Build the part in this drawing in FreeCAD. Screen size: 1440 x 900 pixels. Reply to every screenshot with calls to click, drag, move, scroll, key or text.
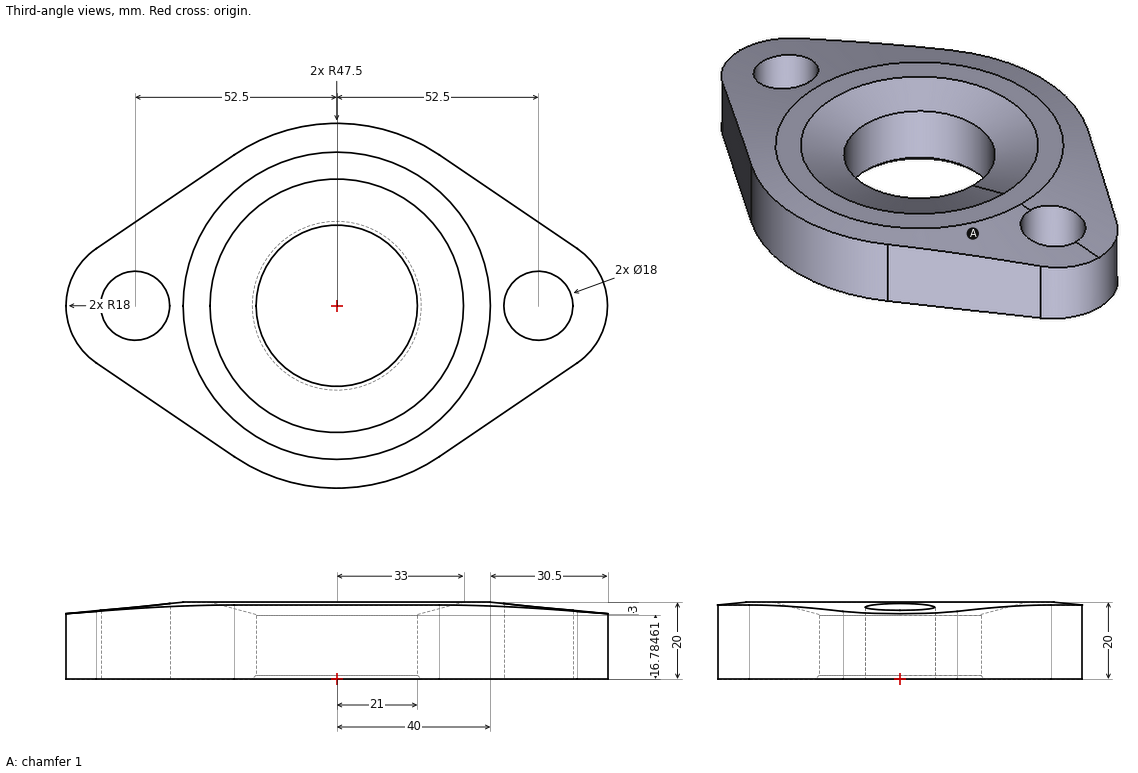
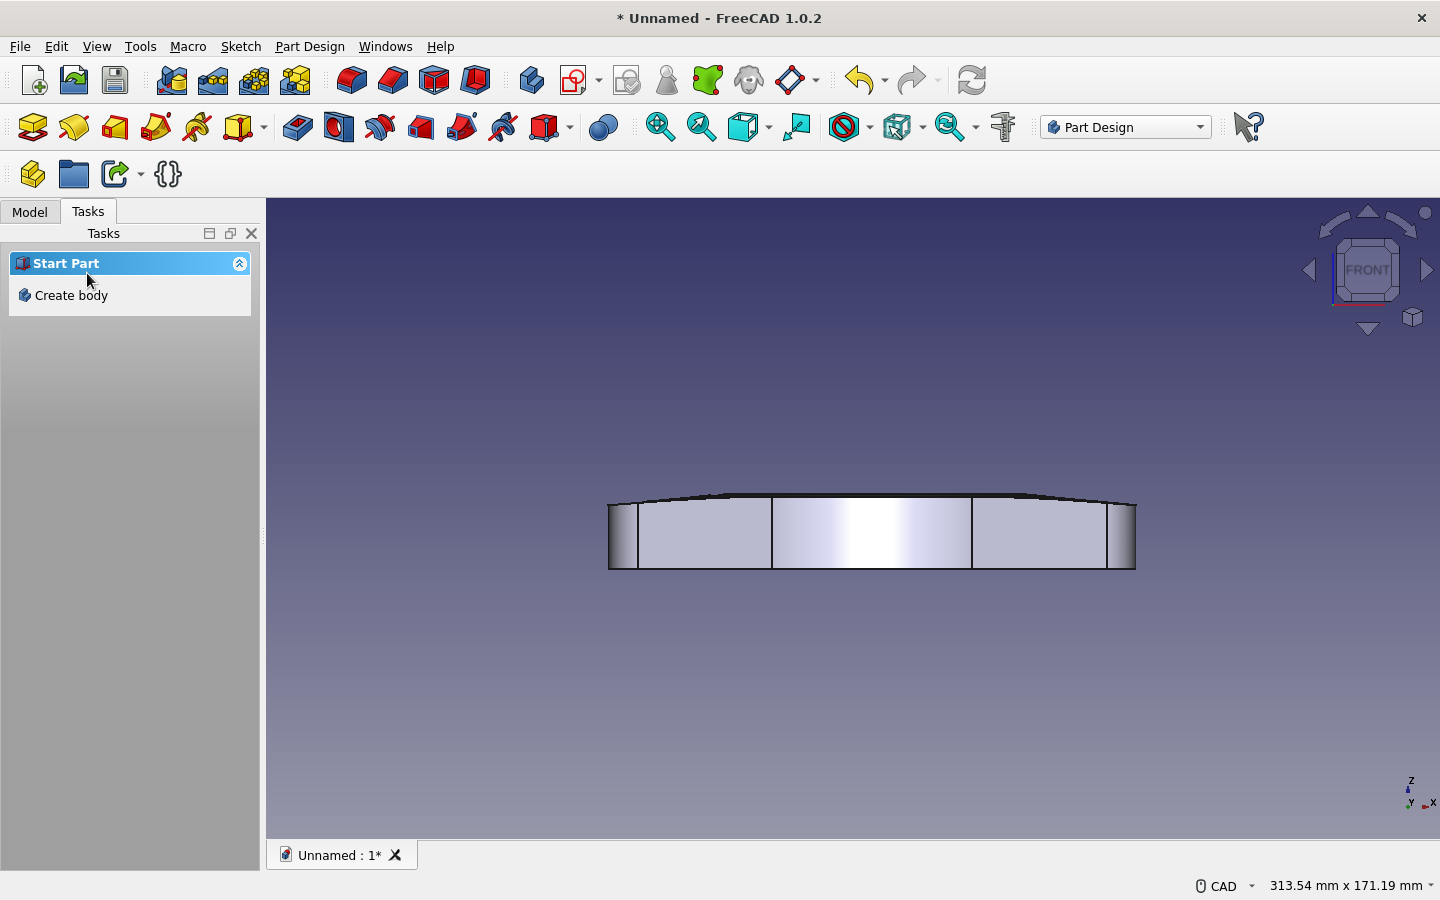
key(v)
key(f)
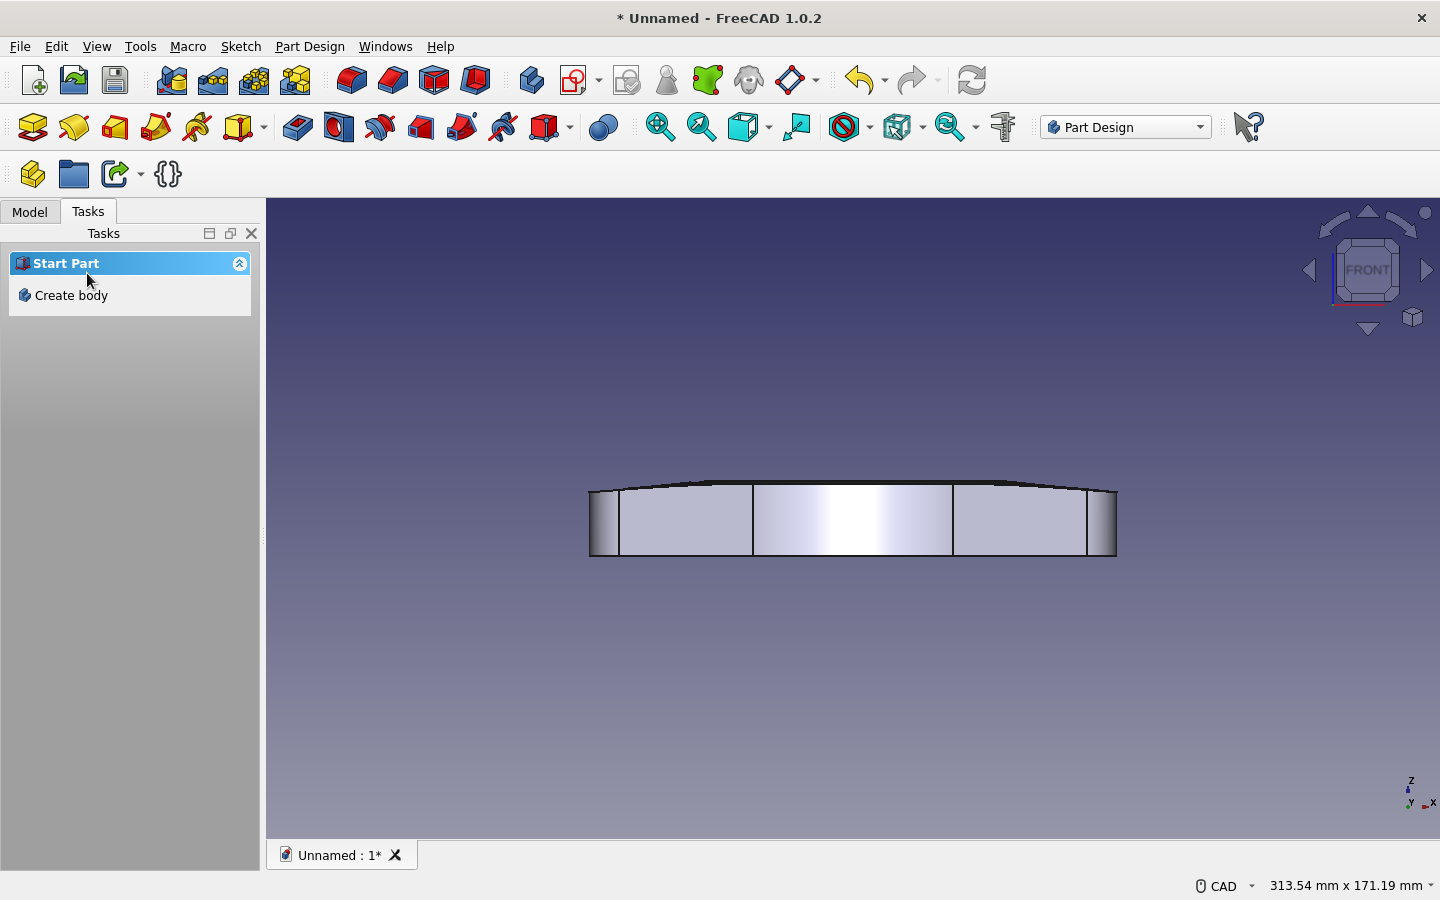
key(3)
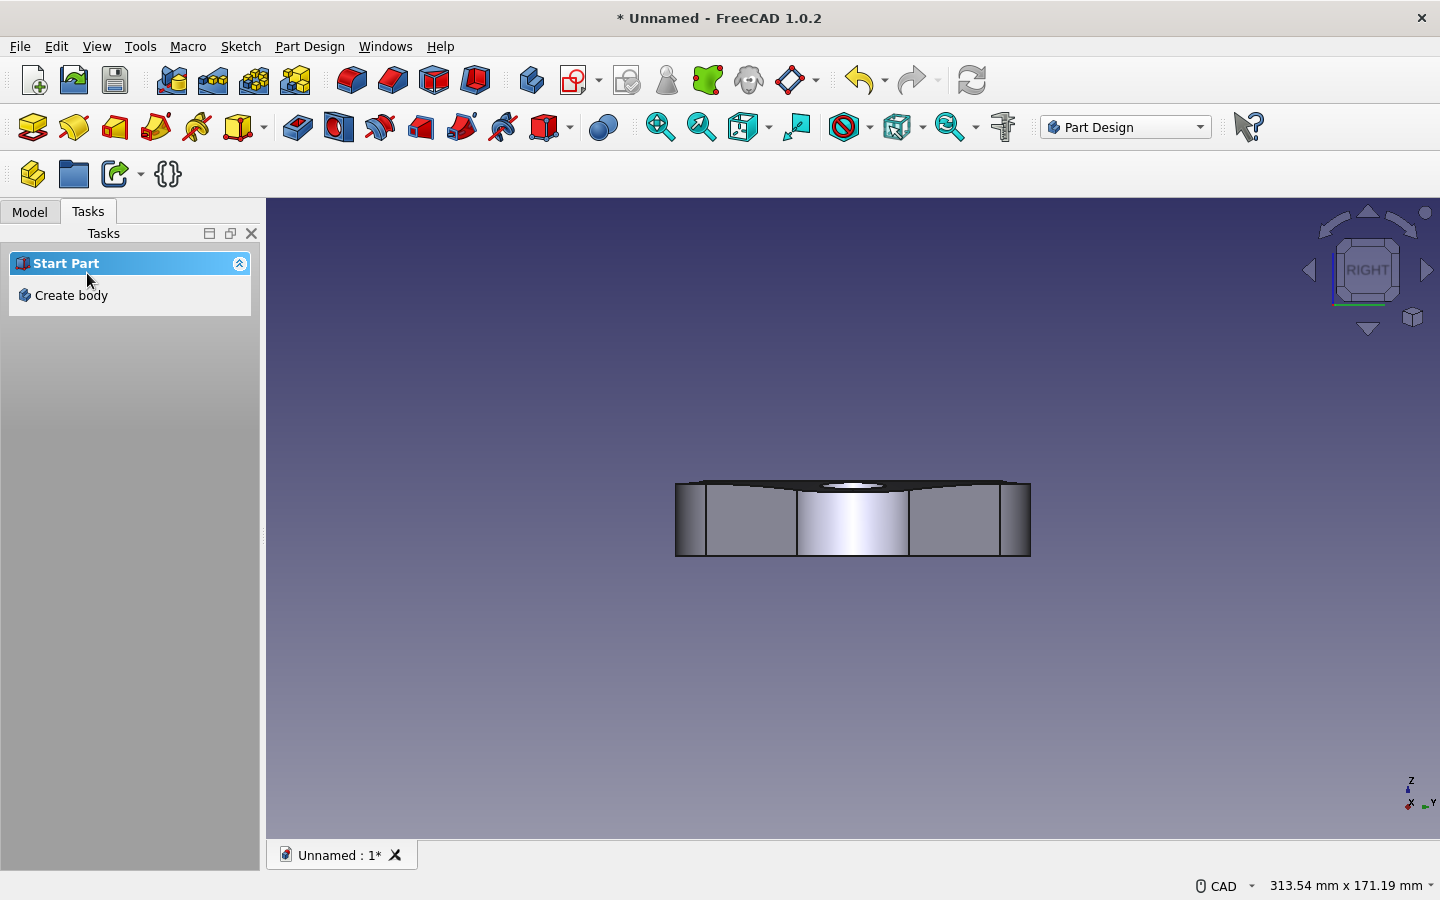
key(v)
key(f)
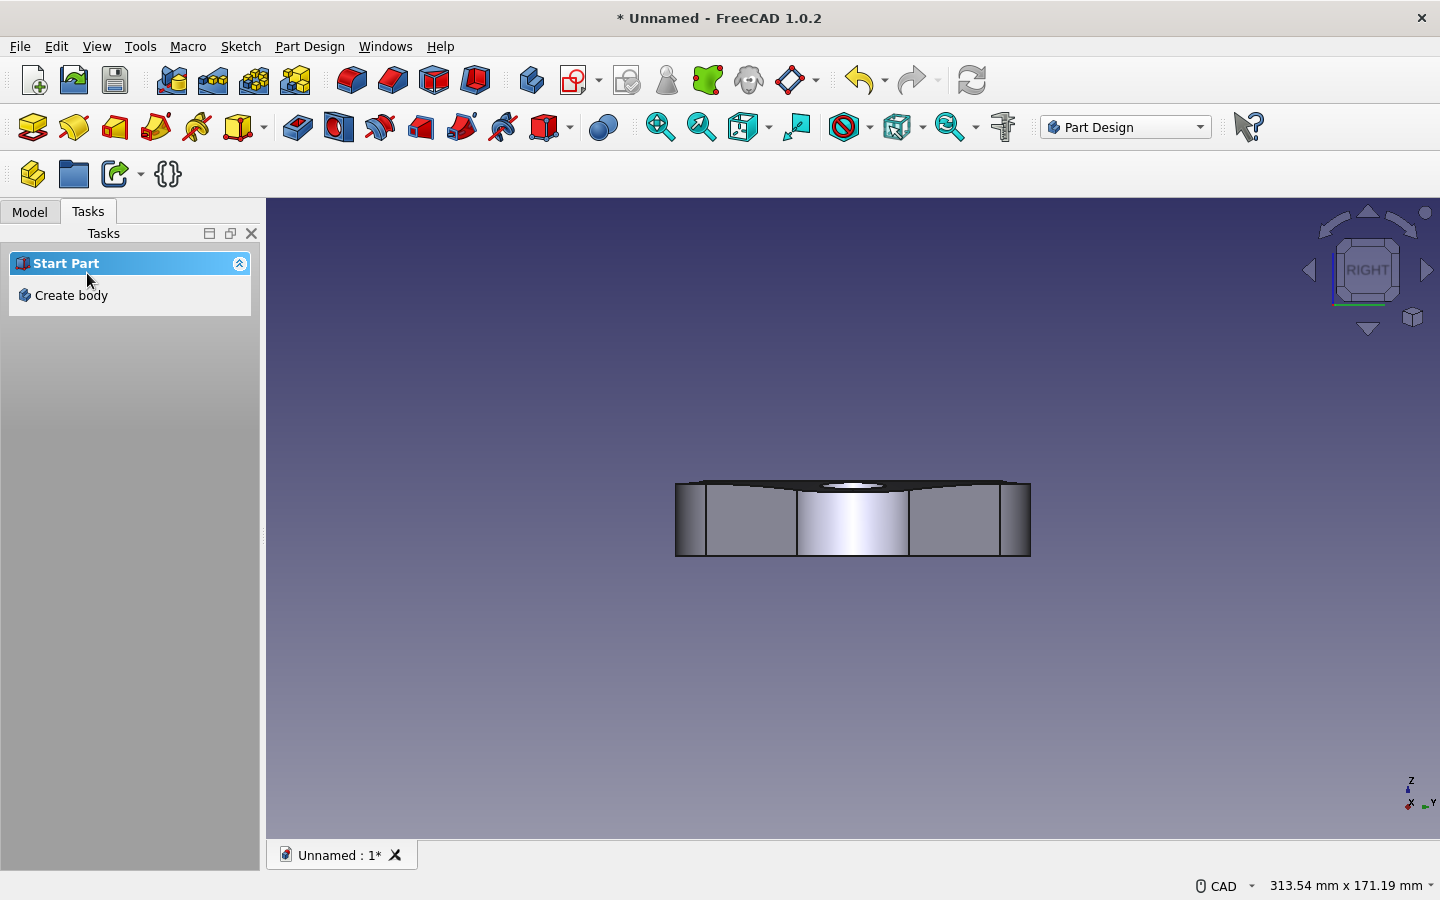
key(5)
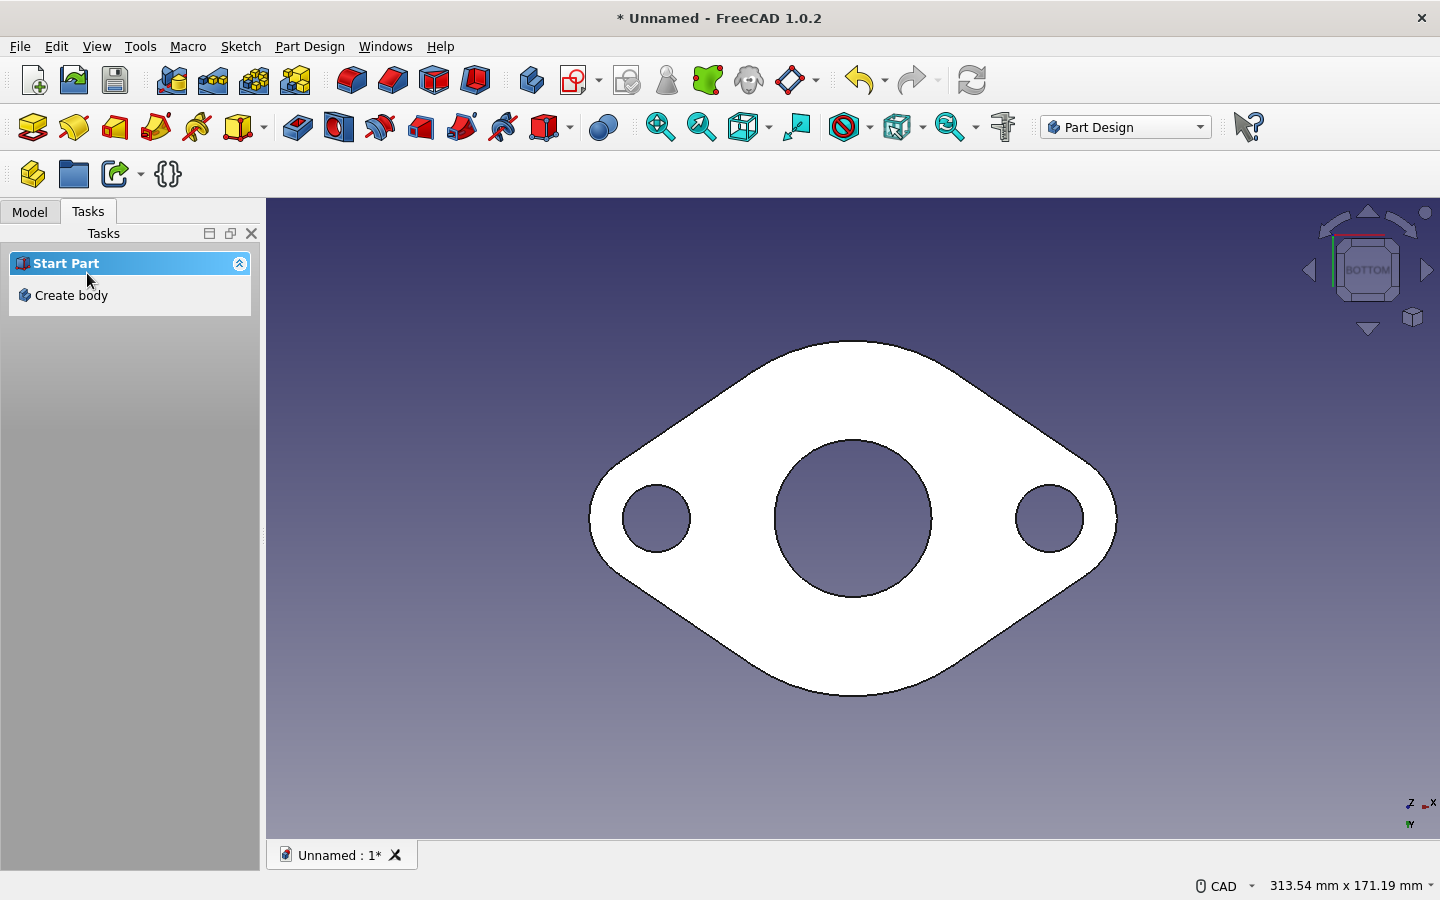
click(774, 517)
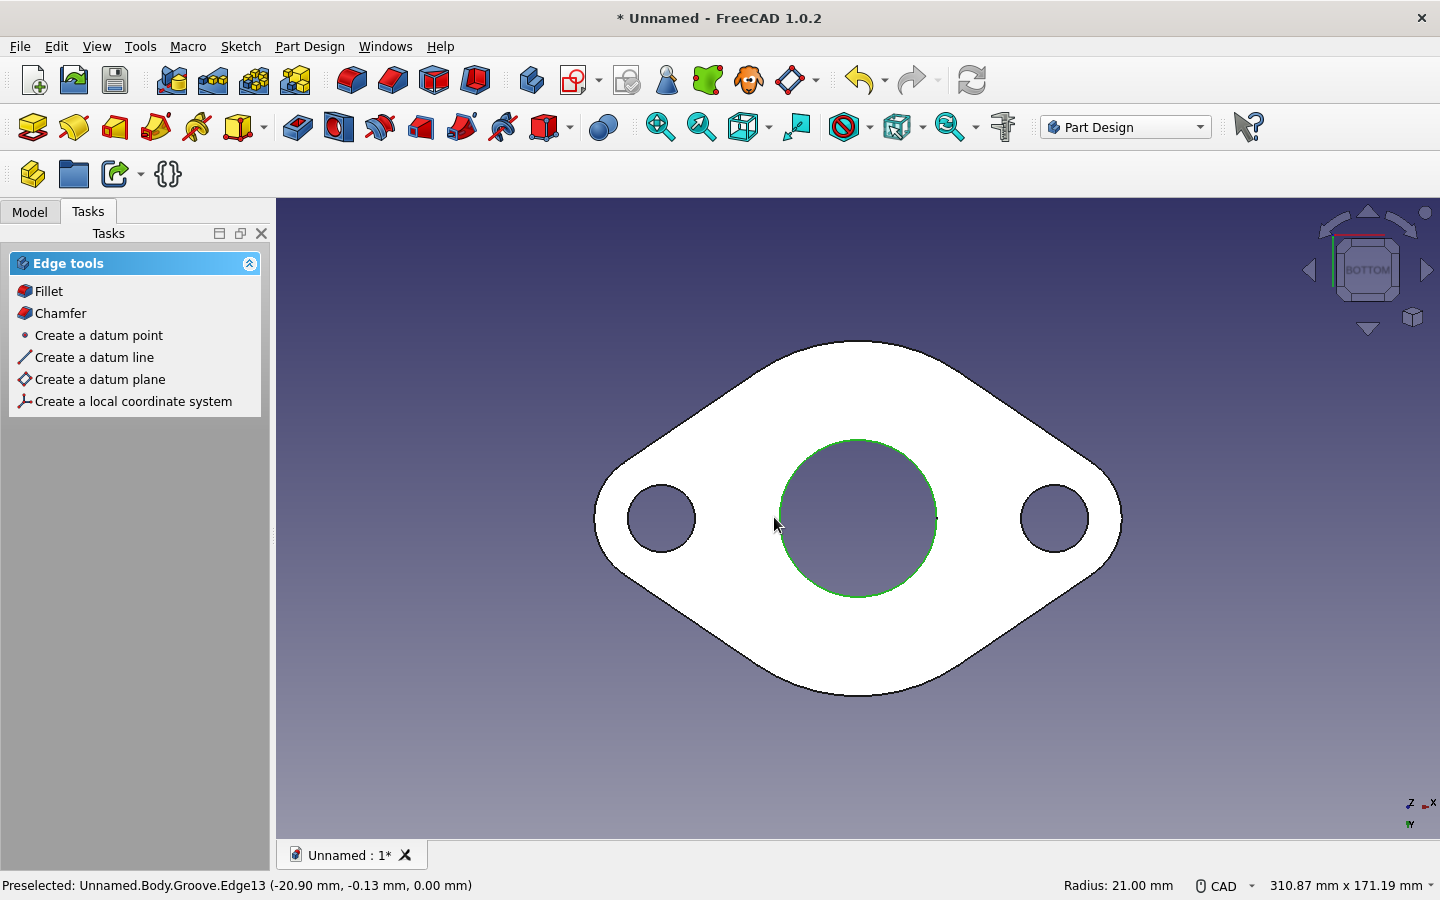
click(393, 80)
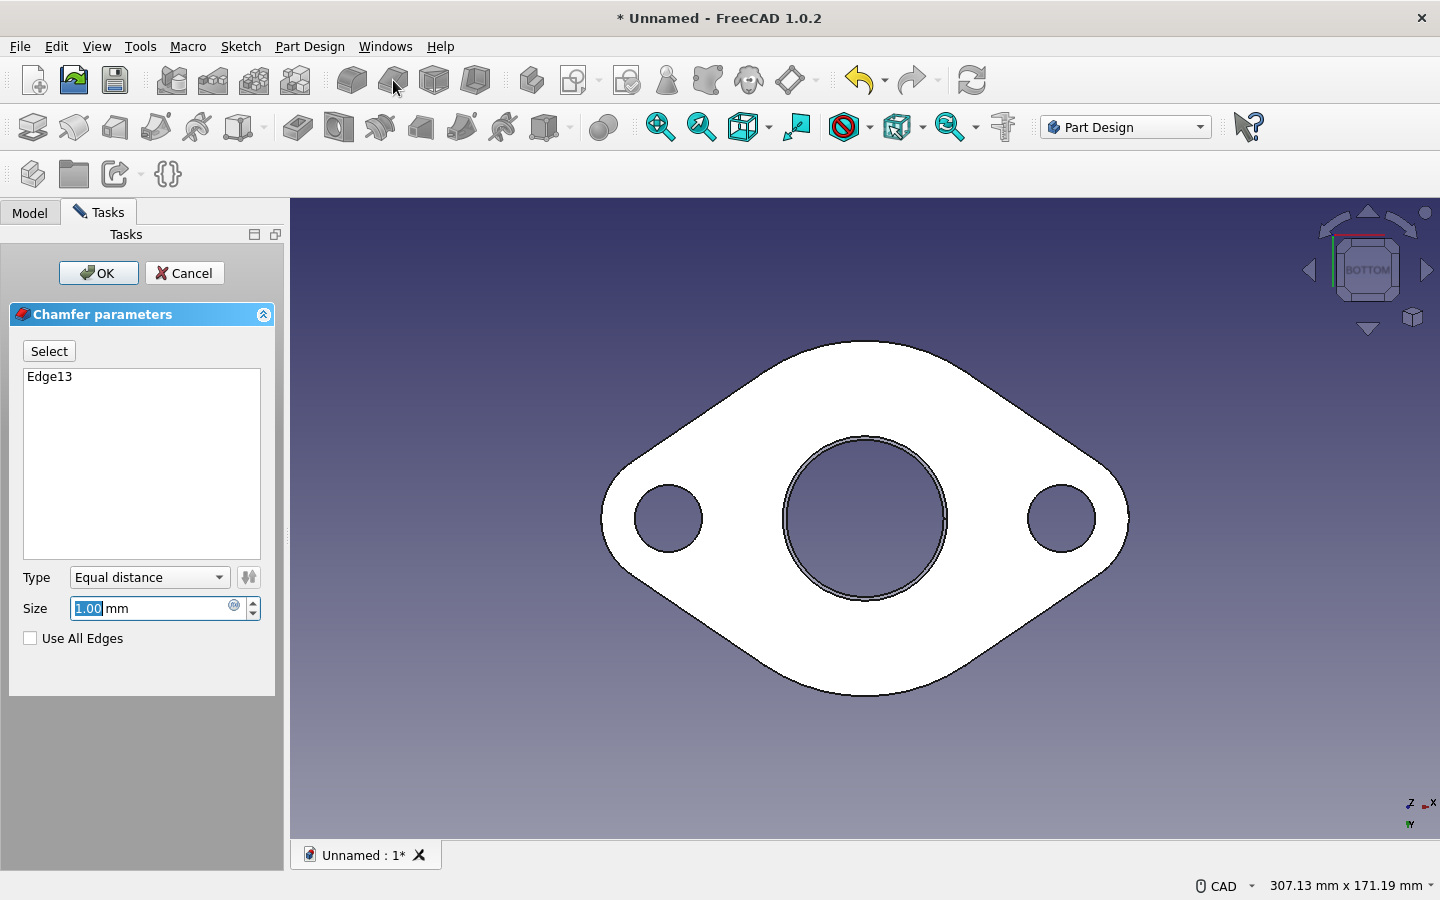
text(1)
key(Tab)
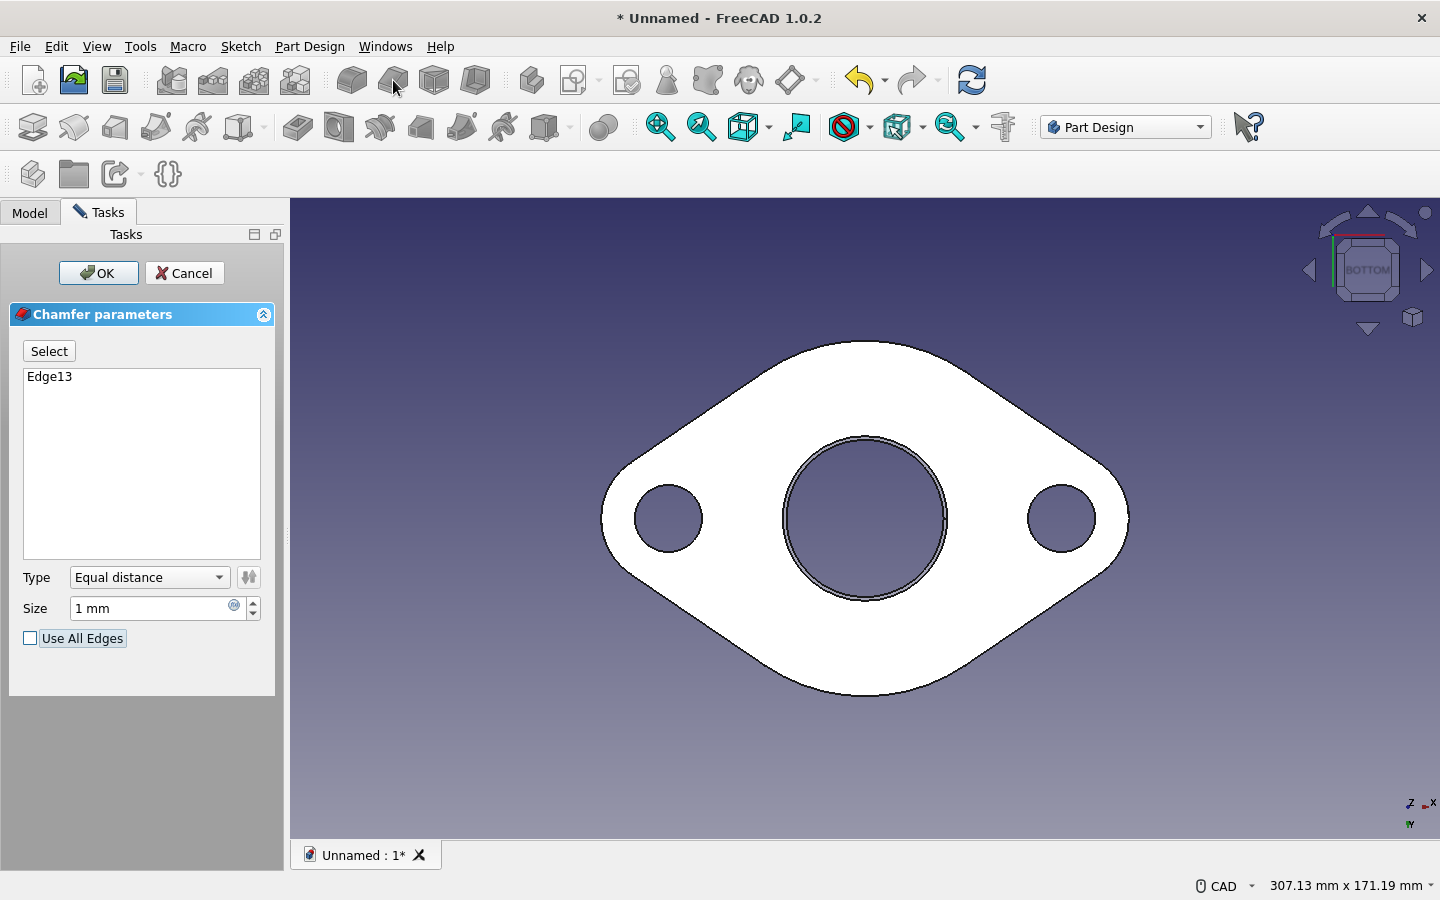
click(99, 273)